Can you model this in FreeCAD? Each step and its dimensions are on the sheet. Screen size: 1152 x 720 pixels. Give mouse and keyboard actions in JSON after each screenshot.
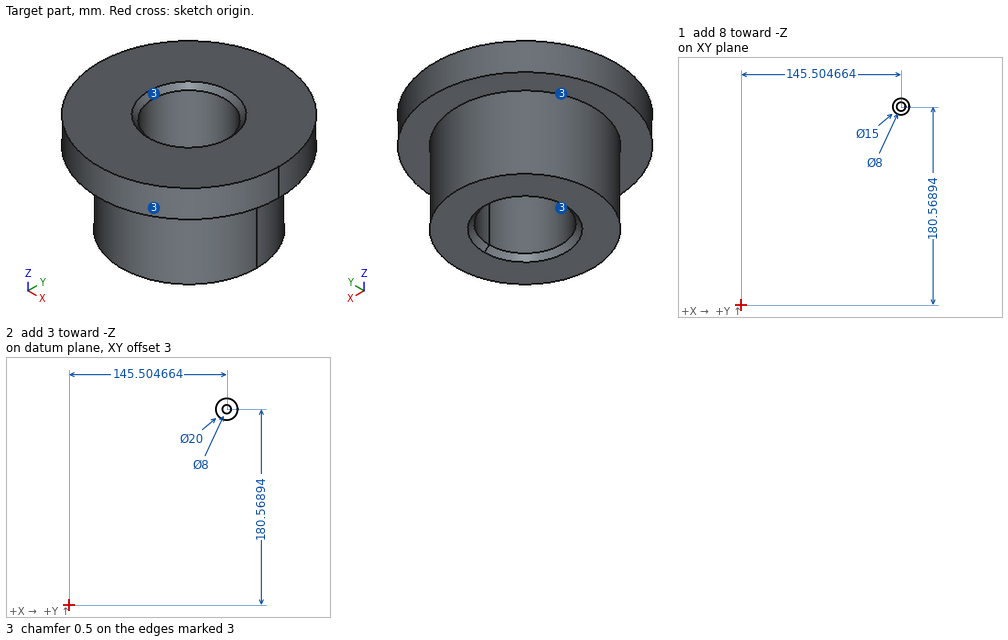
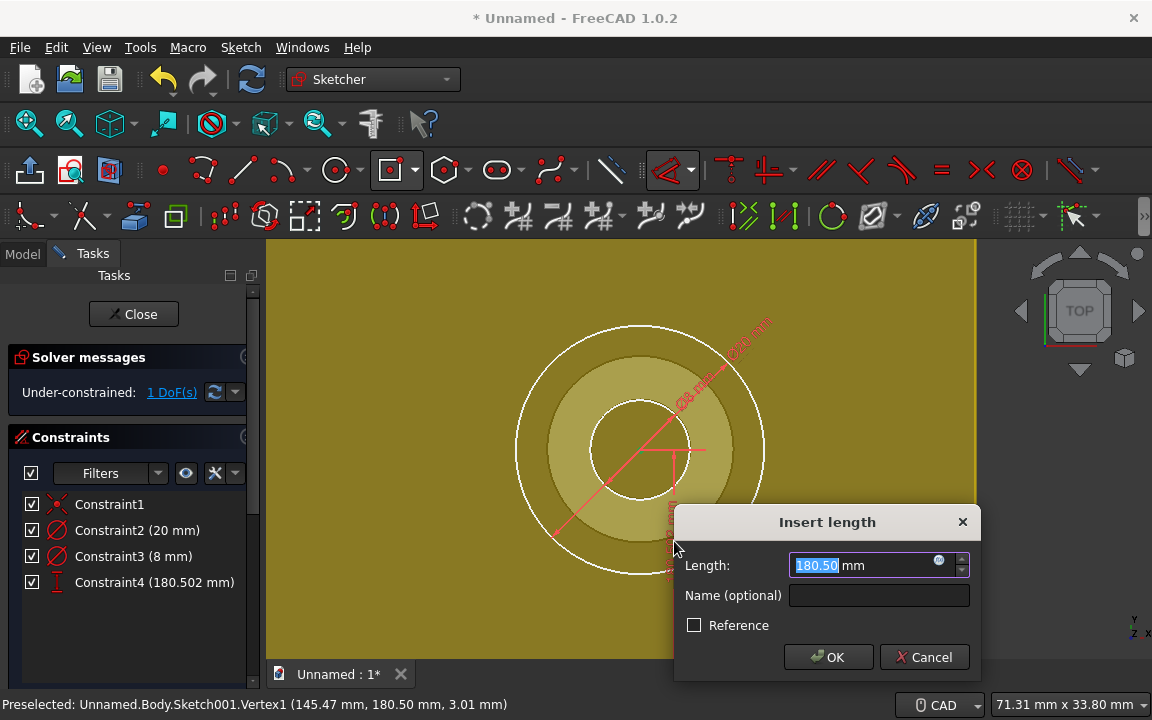
{"action": "type", "text": "180.56894"}
{"action": "key", "text": "Return"}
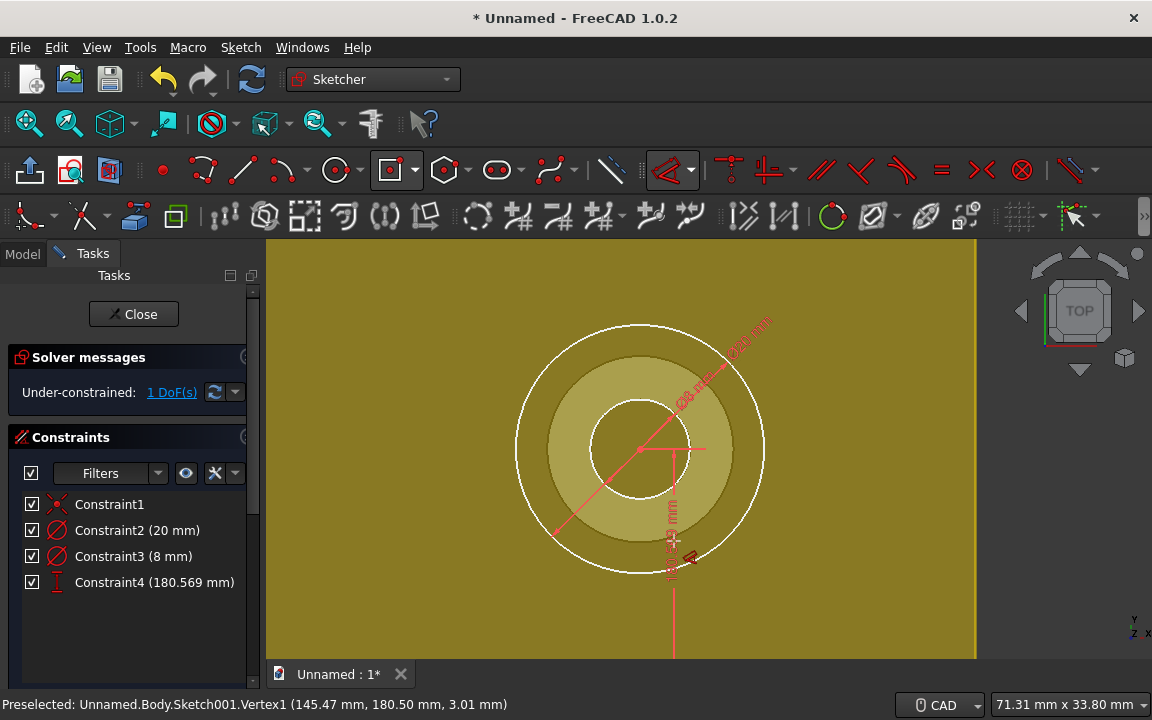
{"action": "left_click", "coordinate": [640, 449]}
{"action": "left_click", "coordinate": [467, 415]}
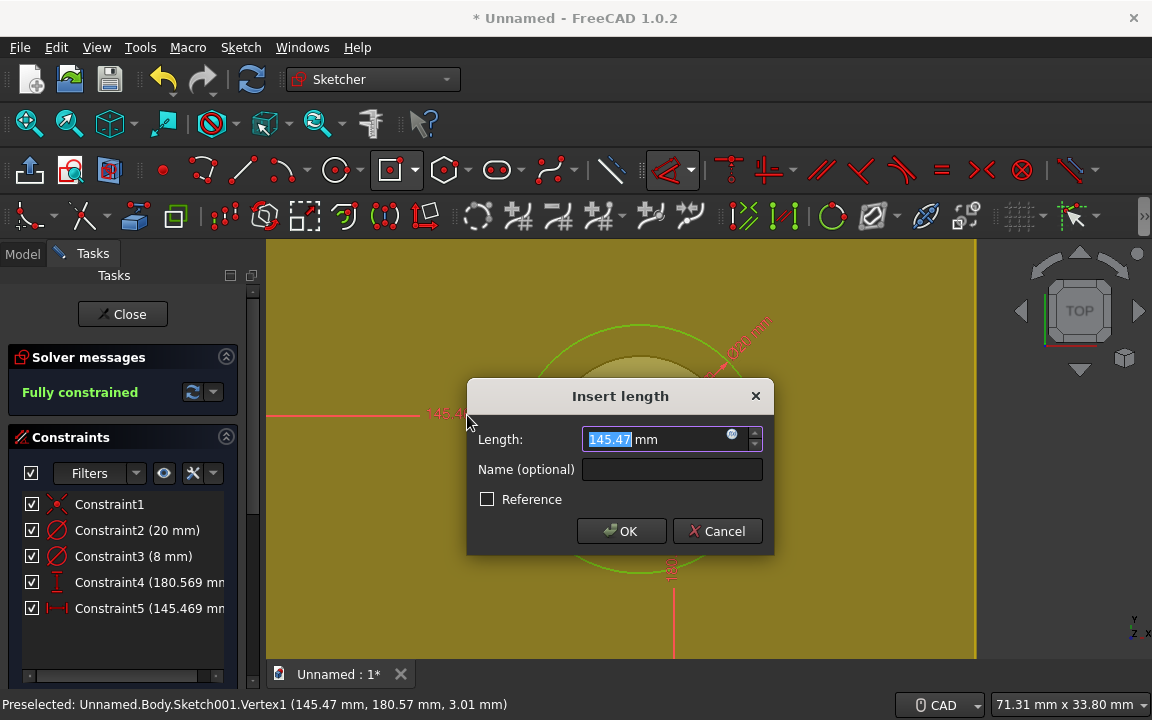
{"action": "type", "text": "145.504664"}
{"action": "key", "text": "Return"}
{"action": "key", "text": "Escape"}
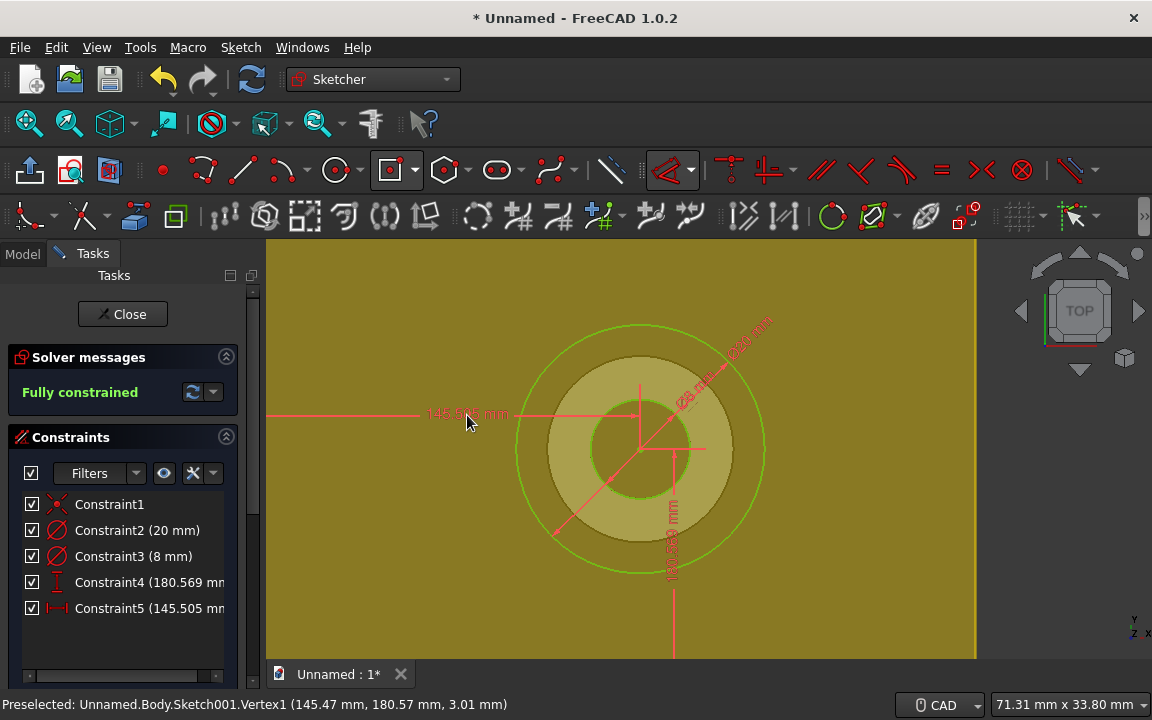
{"action": "left_click", "coordinate": [123, 314]}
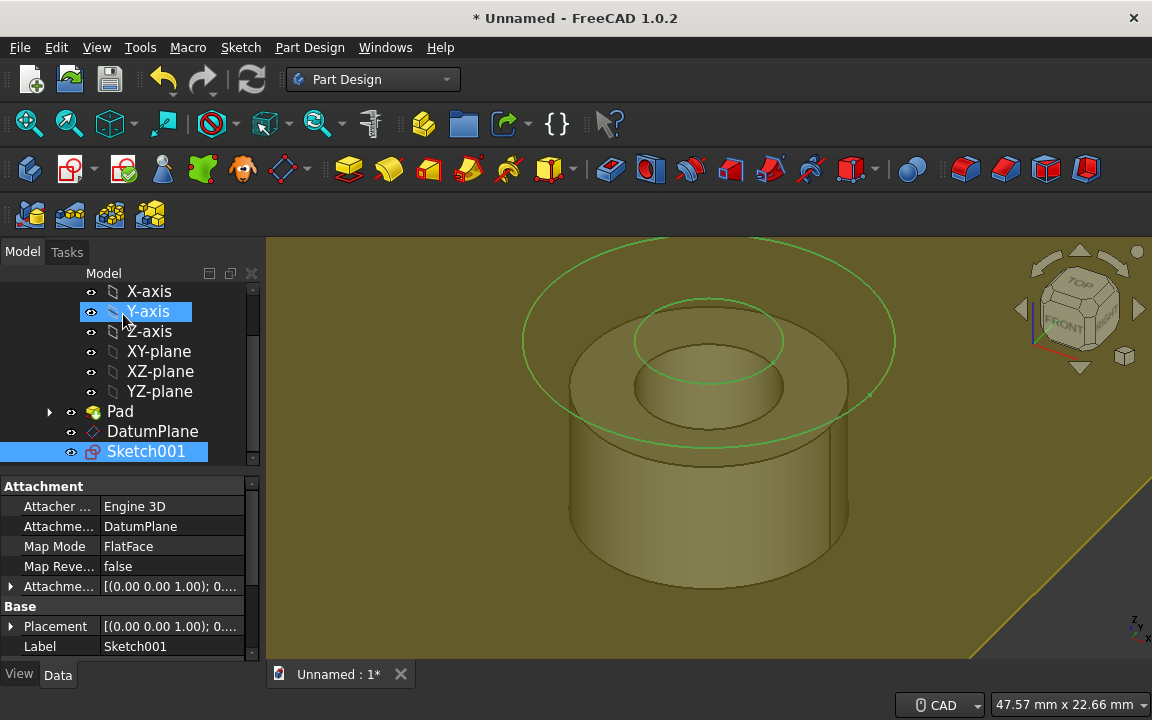
{"action": "left_click", "coordinate": [350, 170]}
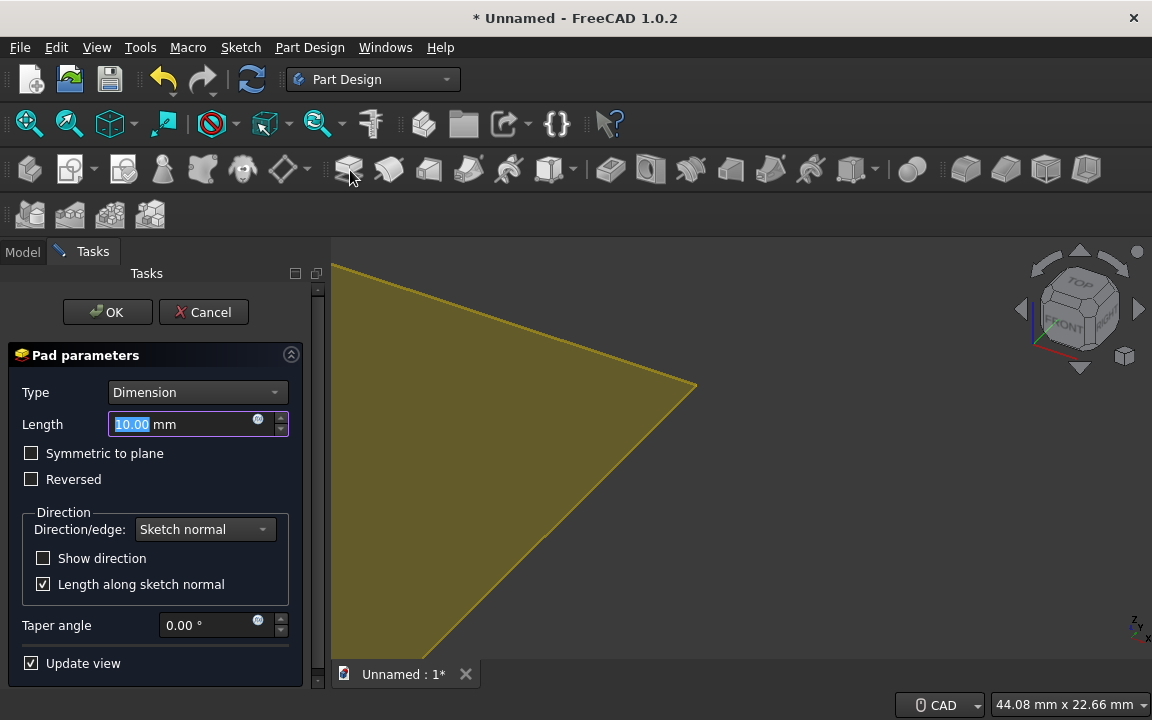
{"action": "type", "text": "3"}
{"action": "key", "text": "Tab"}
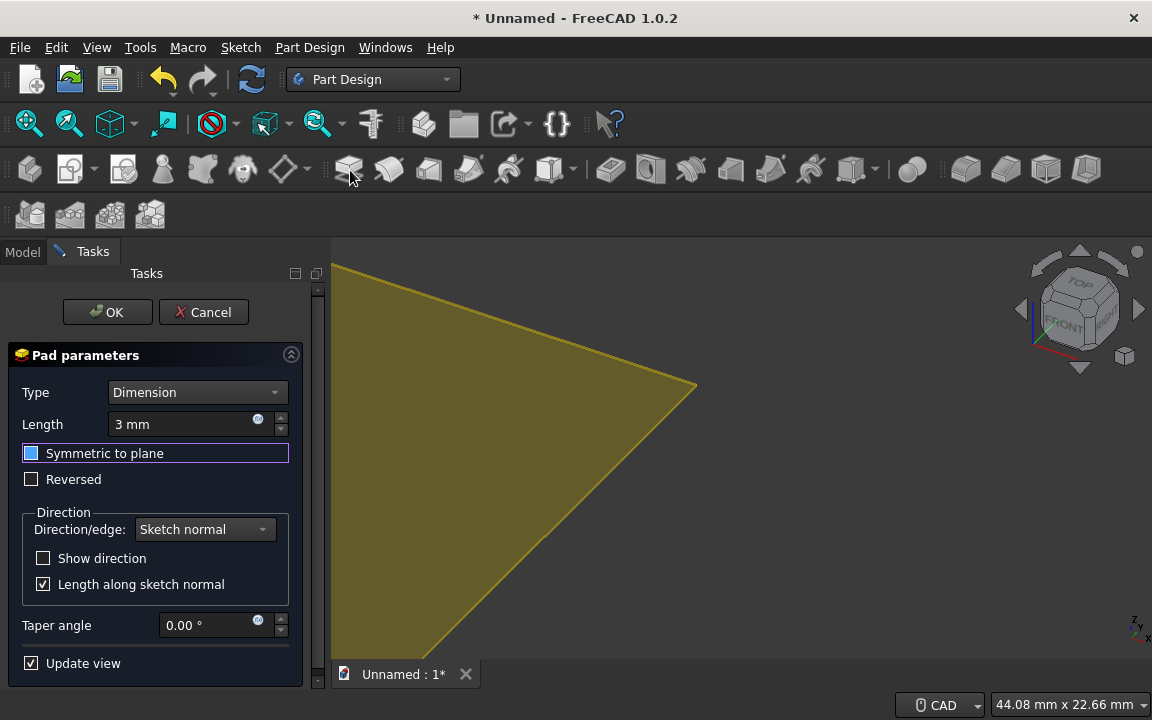
{"action": "left_click", "coordinate": [30, 479]}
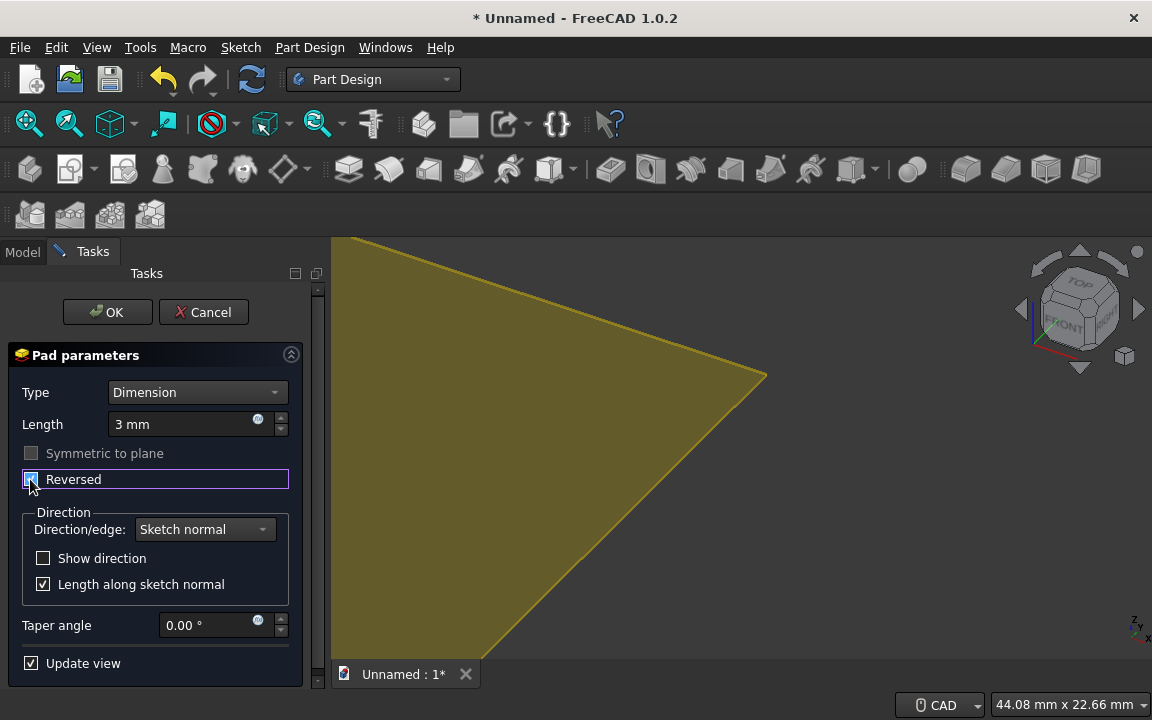
{"action": "left_click", "coordinate": [108, 312]}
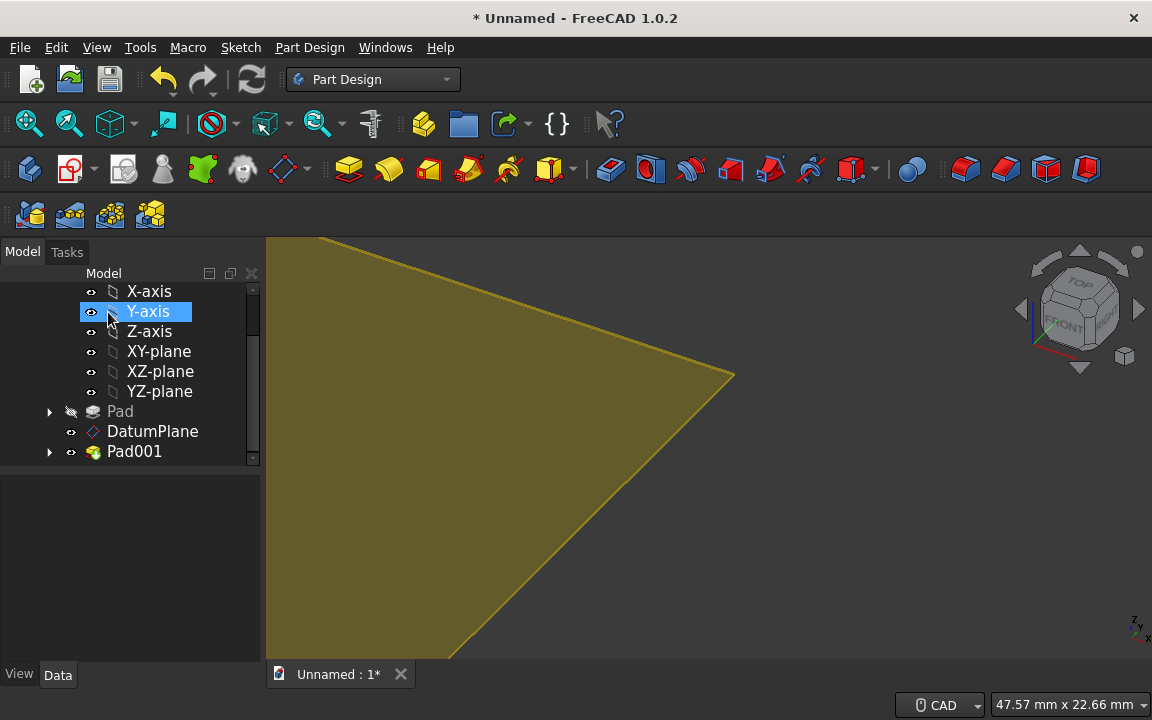
{"action": "left_click", "coordinate": [116, 432]}
{"action": "key", "text": "space"}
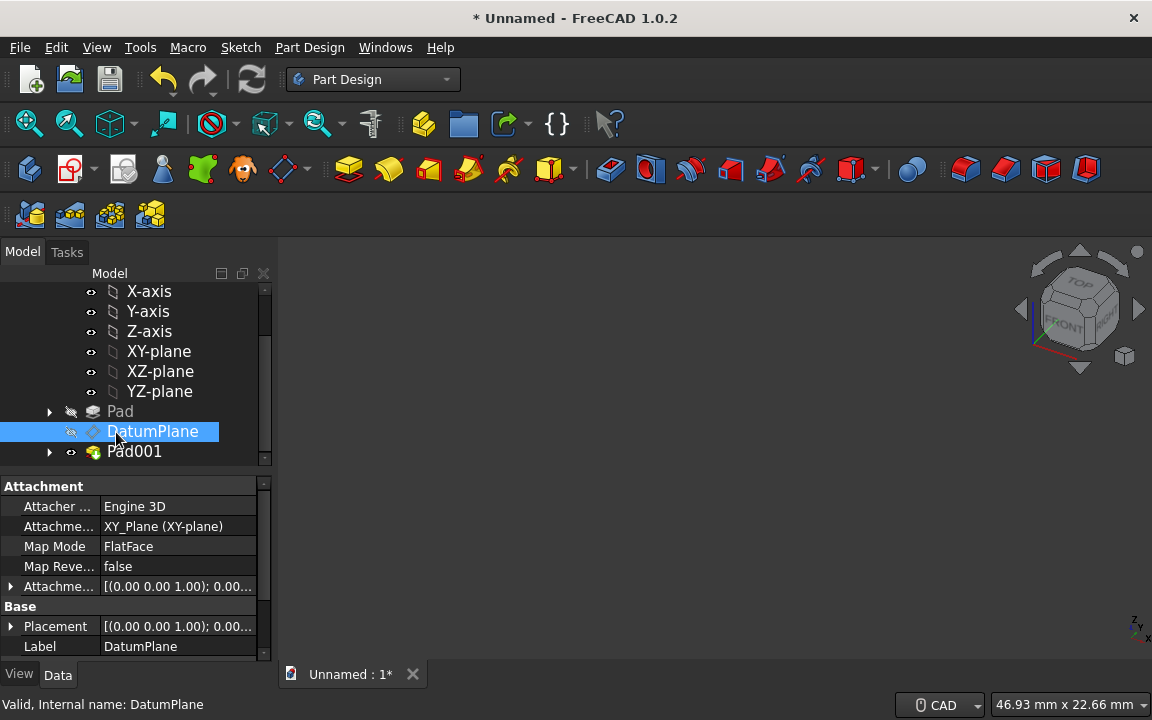
{"action": "key", "text": "v f"}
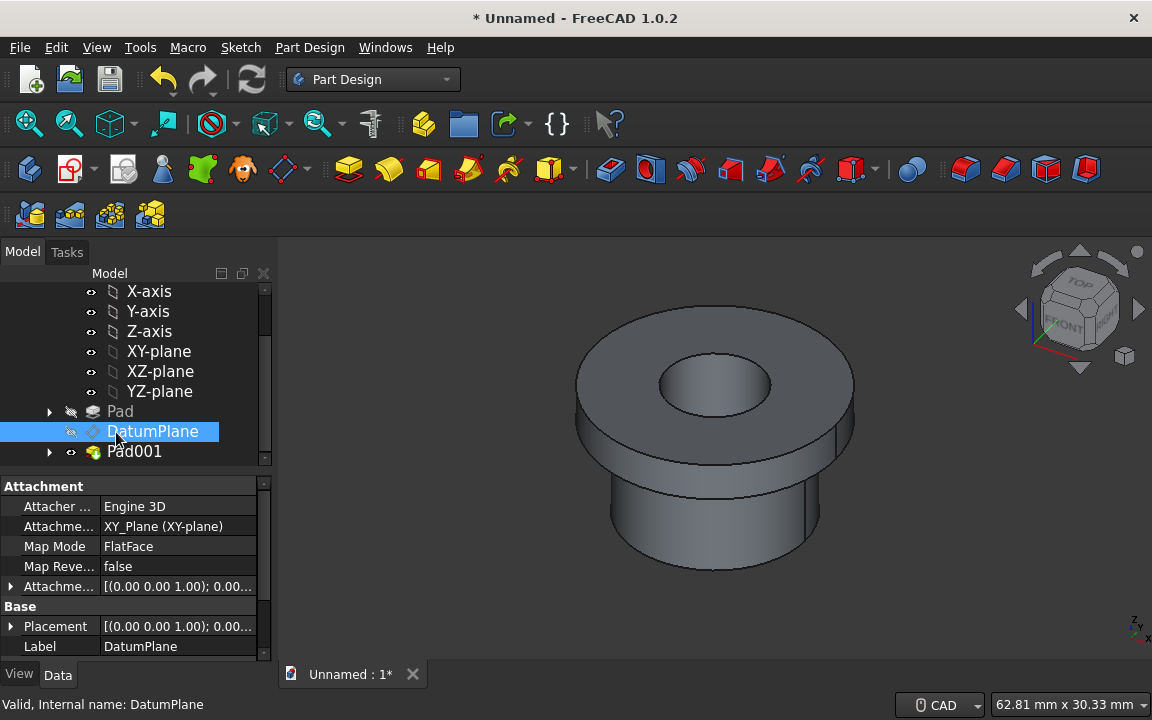
{"action": "left_click", "coordinate": [667, 368]}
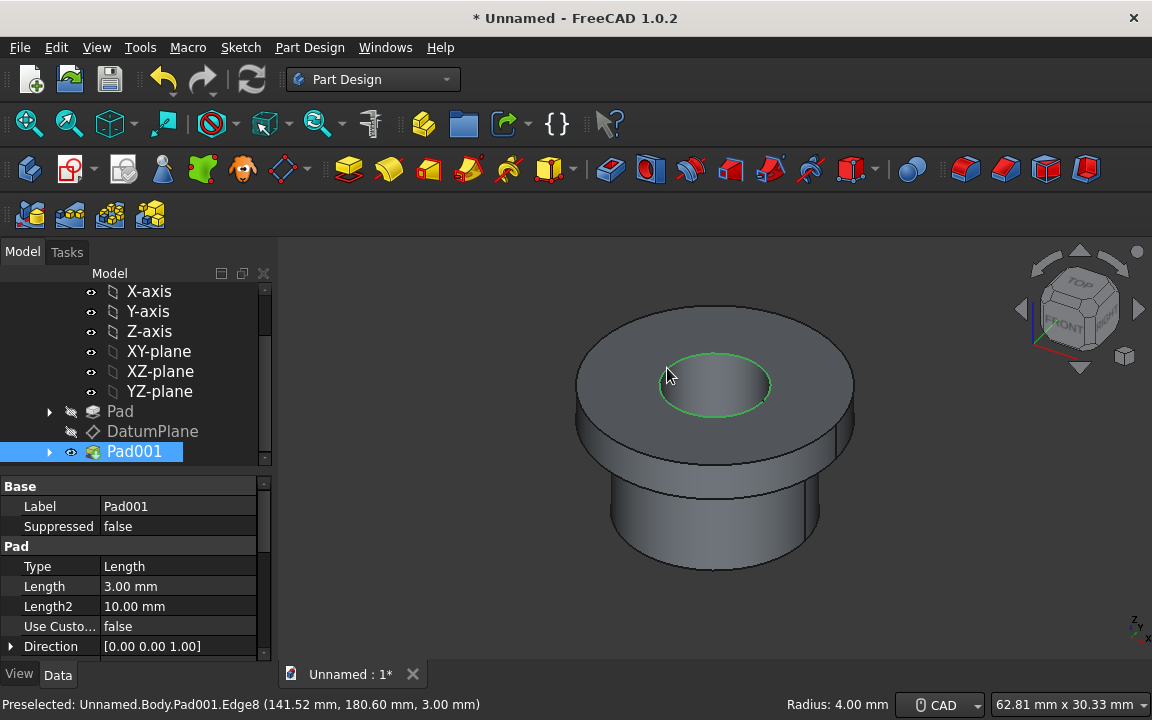
{"action": "key", "text": "0"}